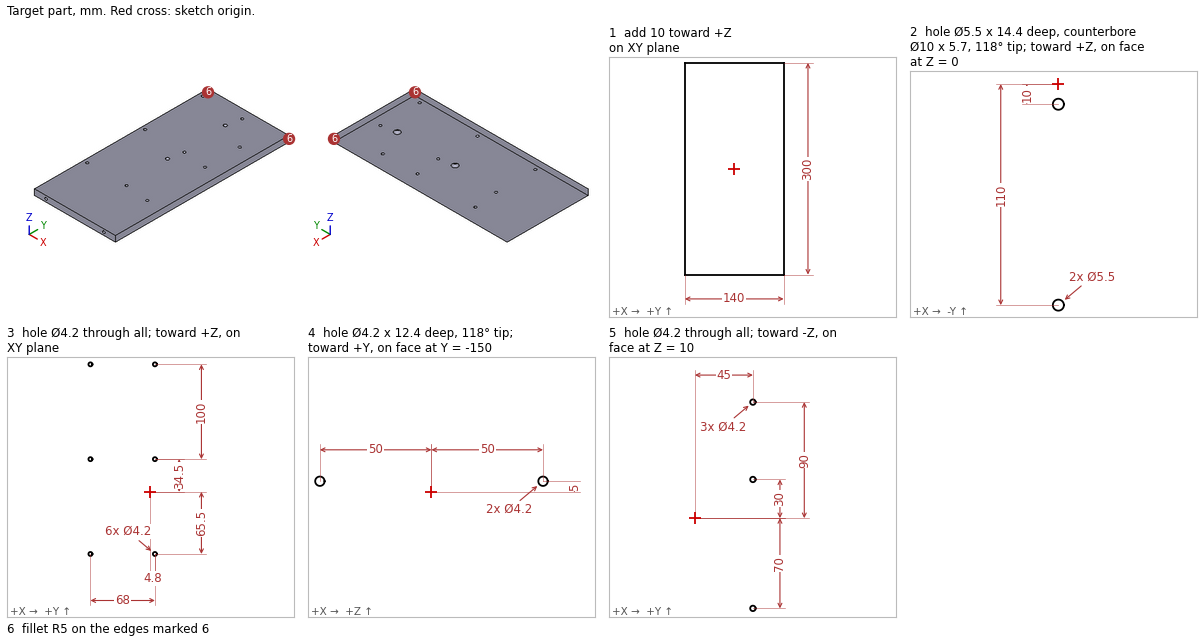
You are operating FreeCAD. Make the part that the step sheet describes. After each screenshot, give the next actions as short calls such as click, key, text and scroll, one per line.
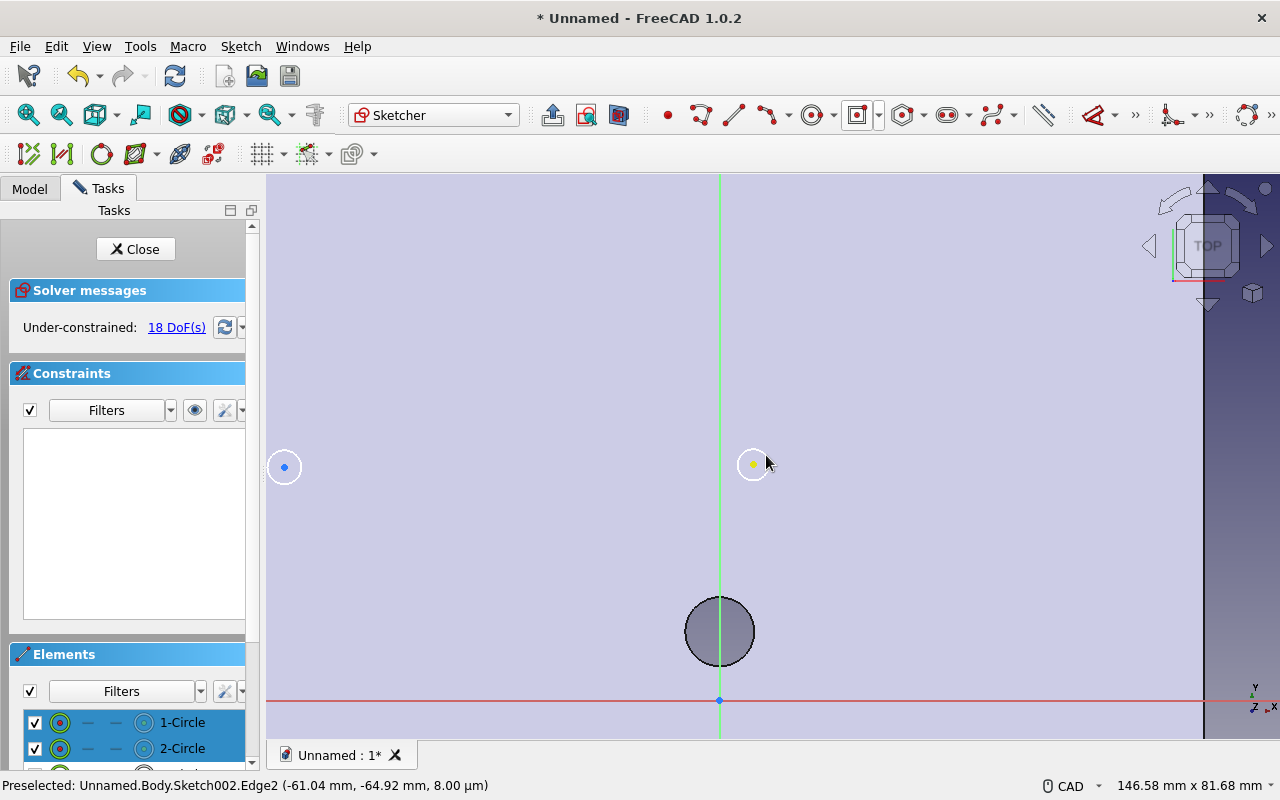
click(764, 454)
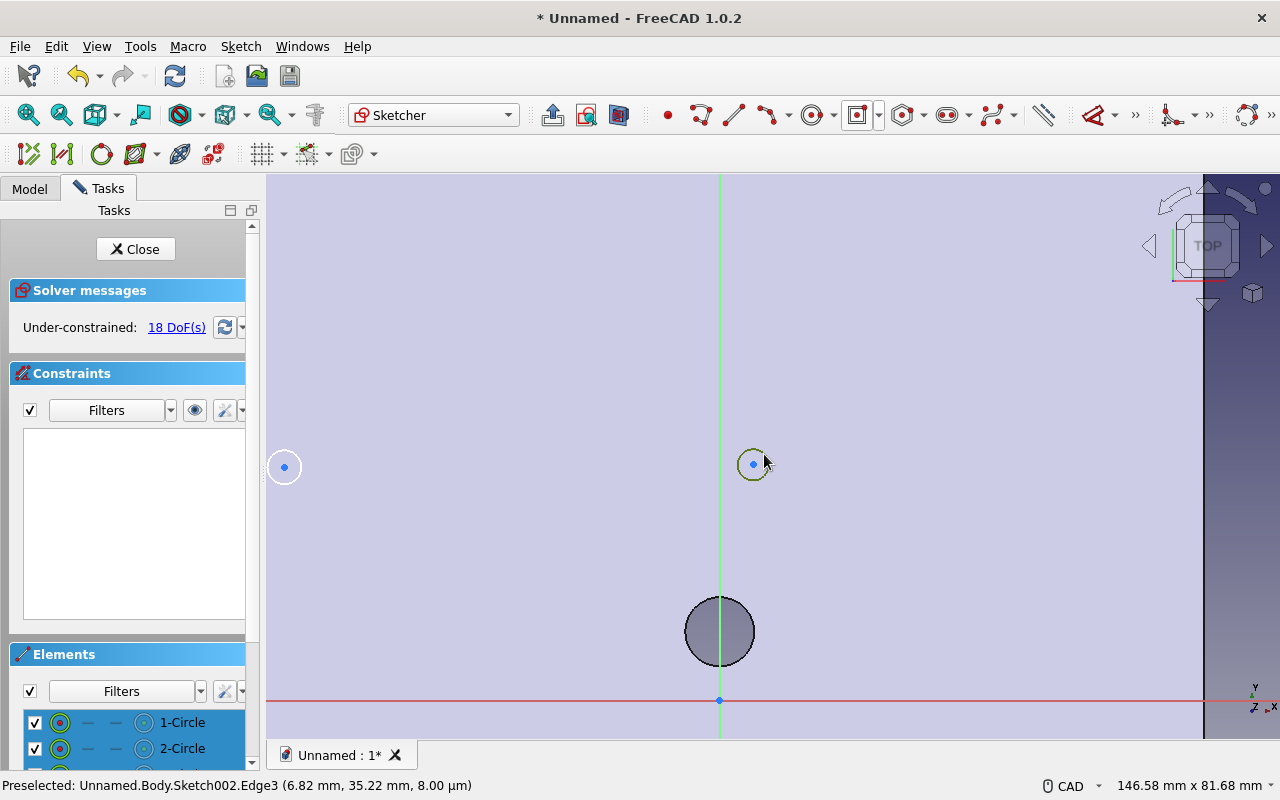
click(296, 455)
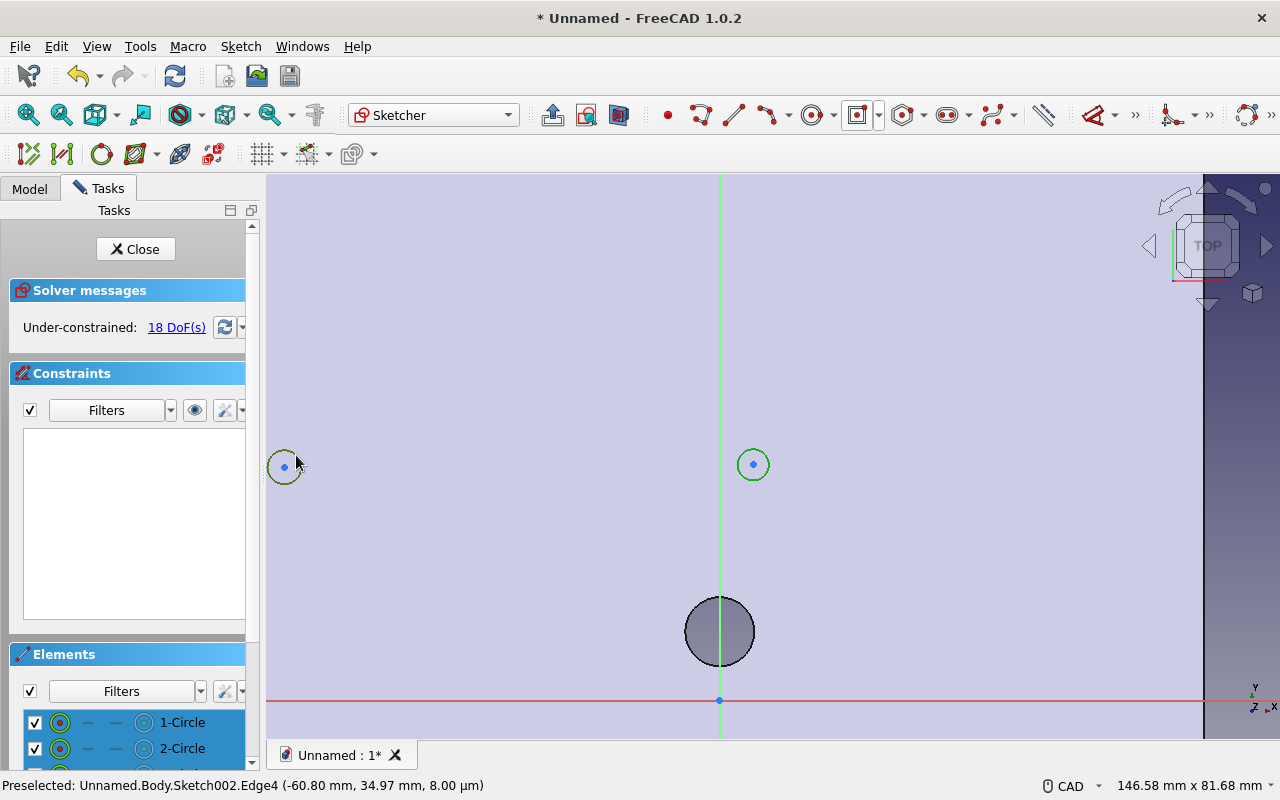
scroll(766, 455, down, 7)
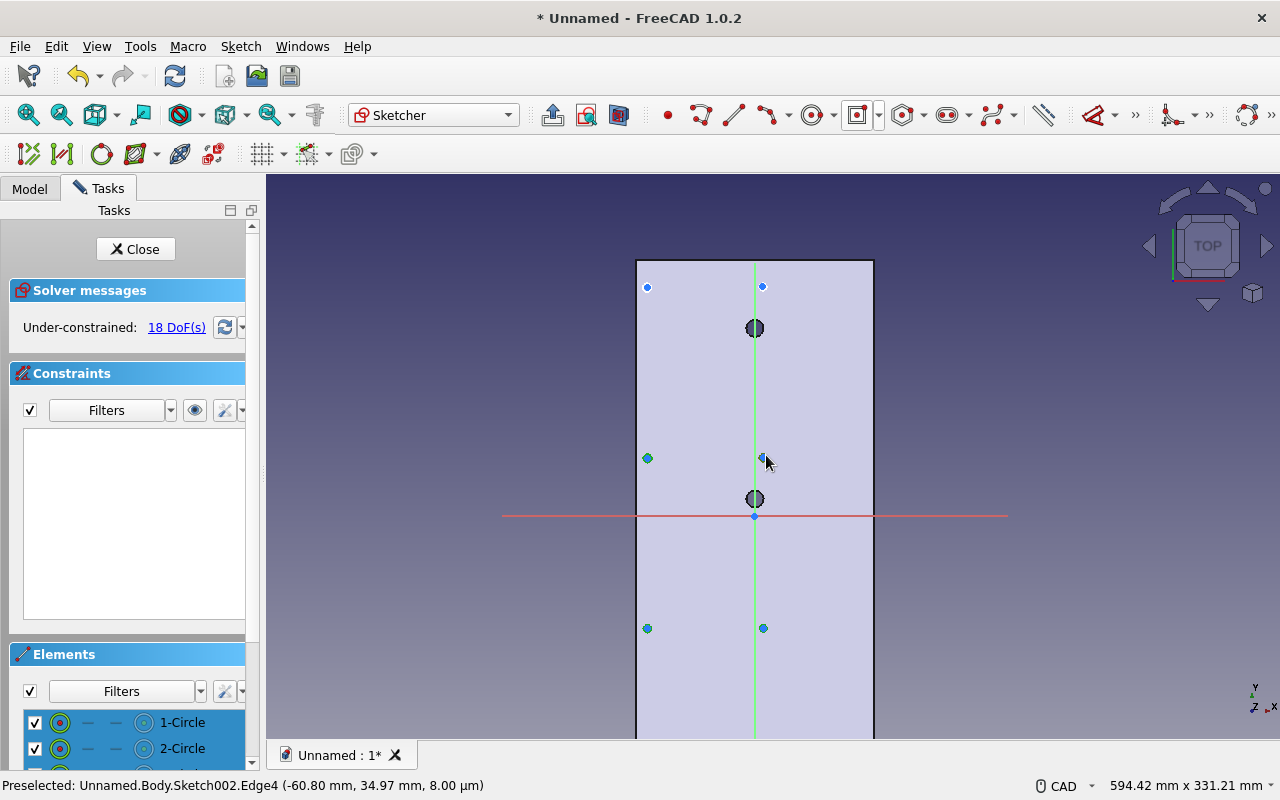
scroll(766, 284, up, 7)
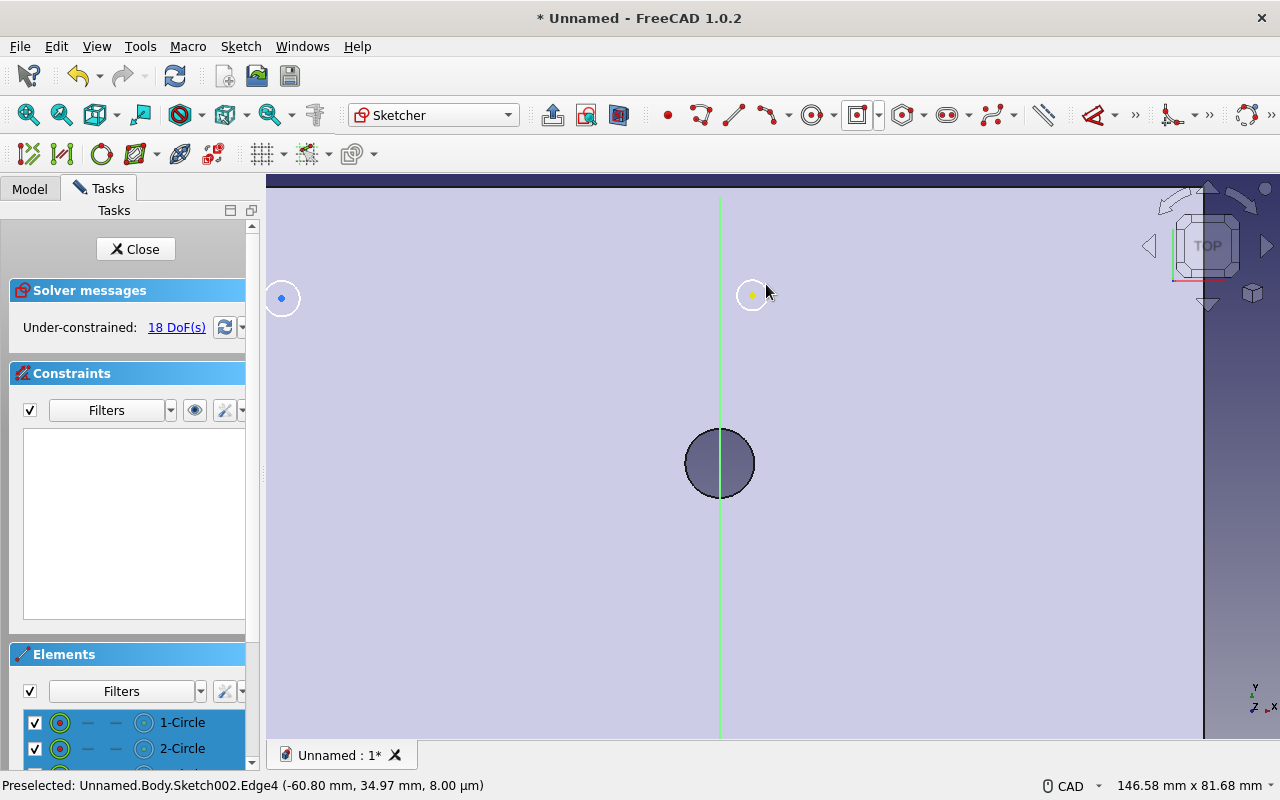
click(763, 285)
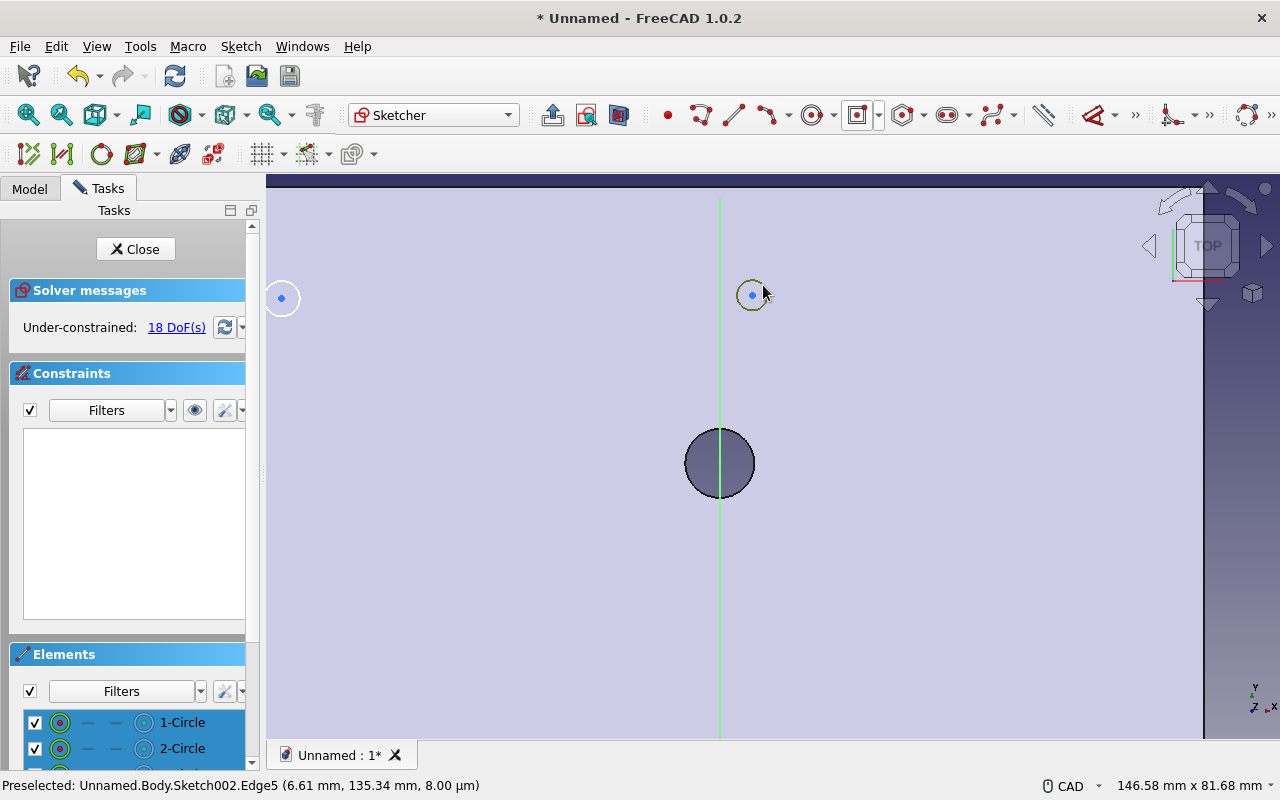
click(294, 286)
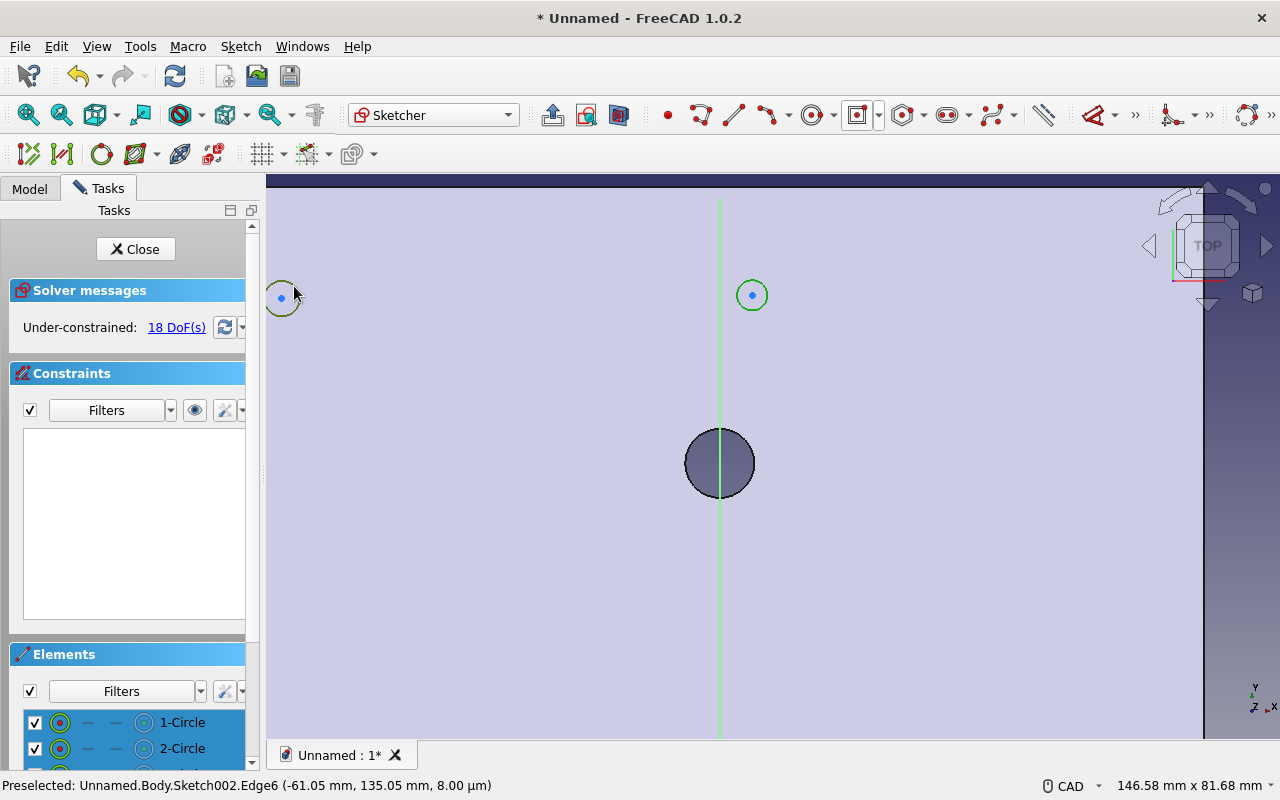
key(e)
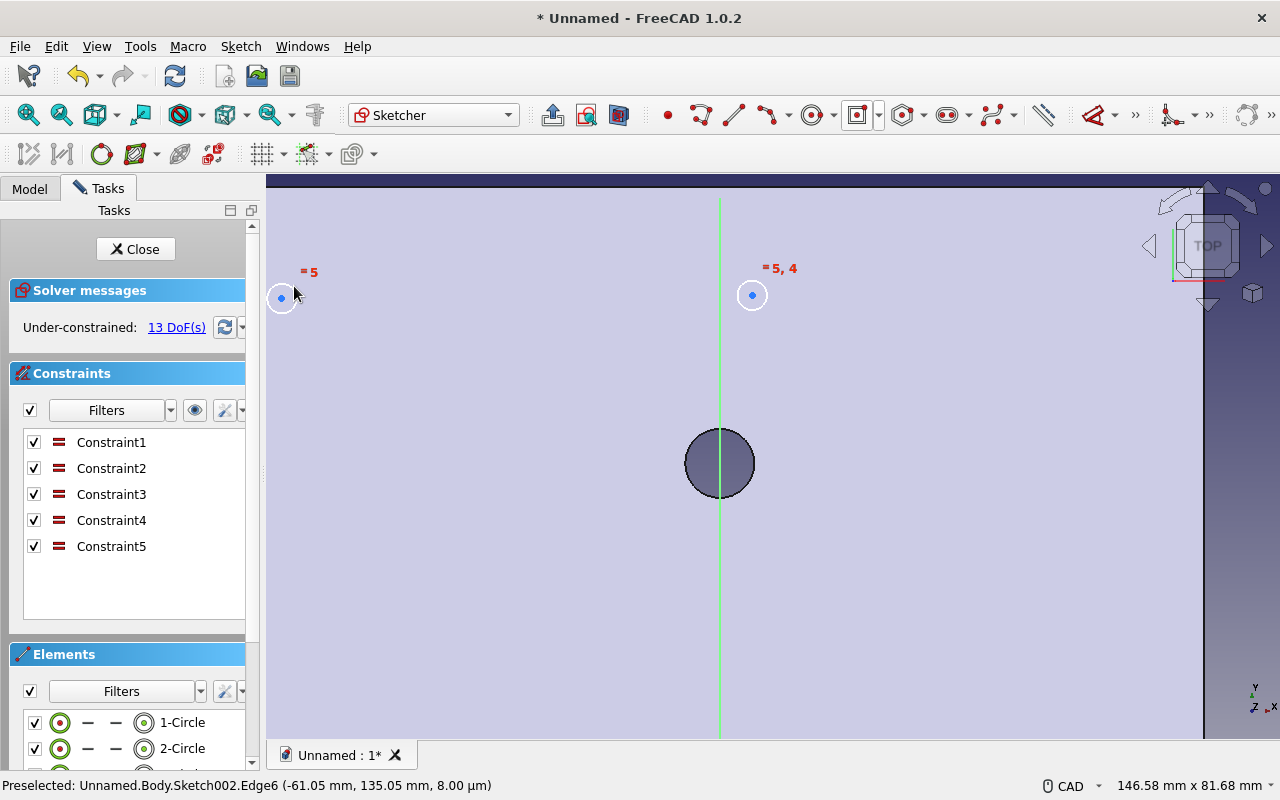
scroll(766, 283, down, 7)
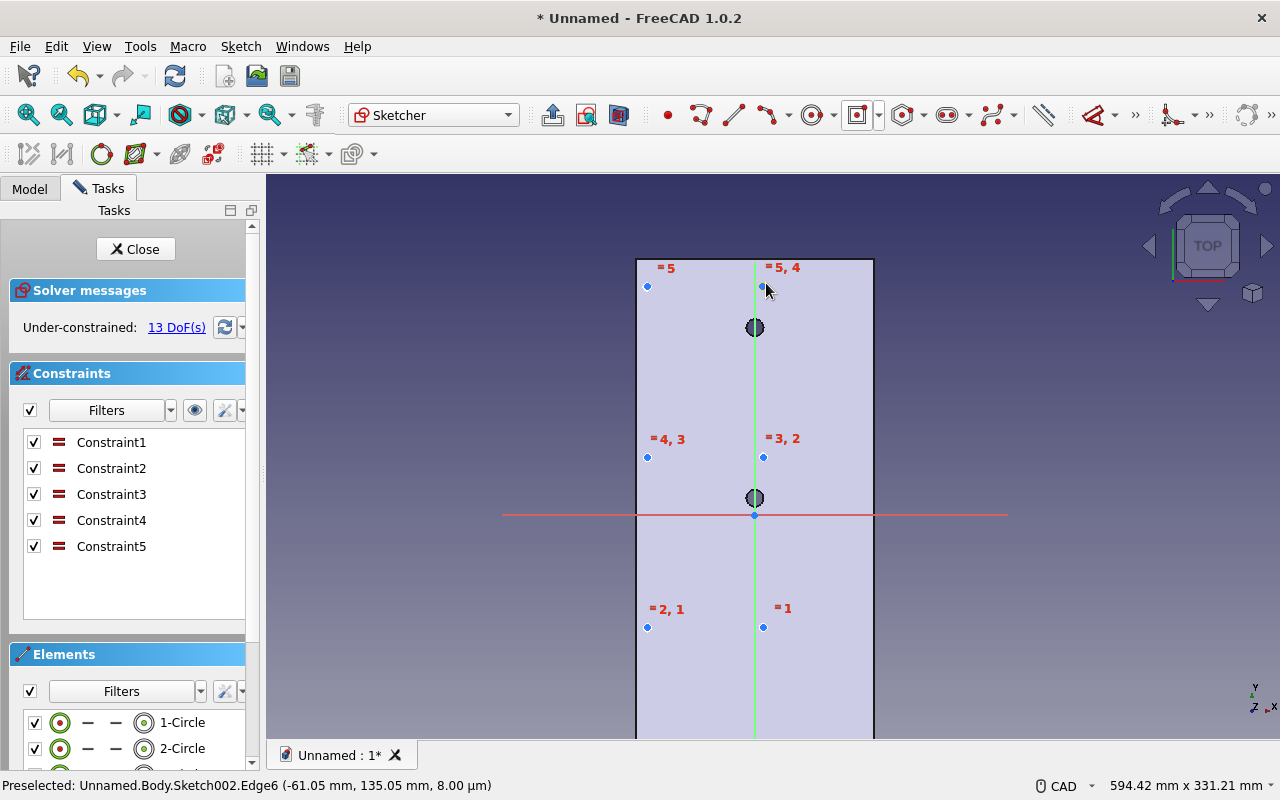
click(763, 627)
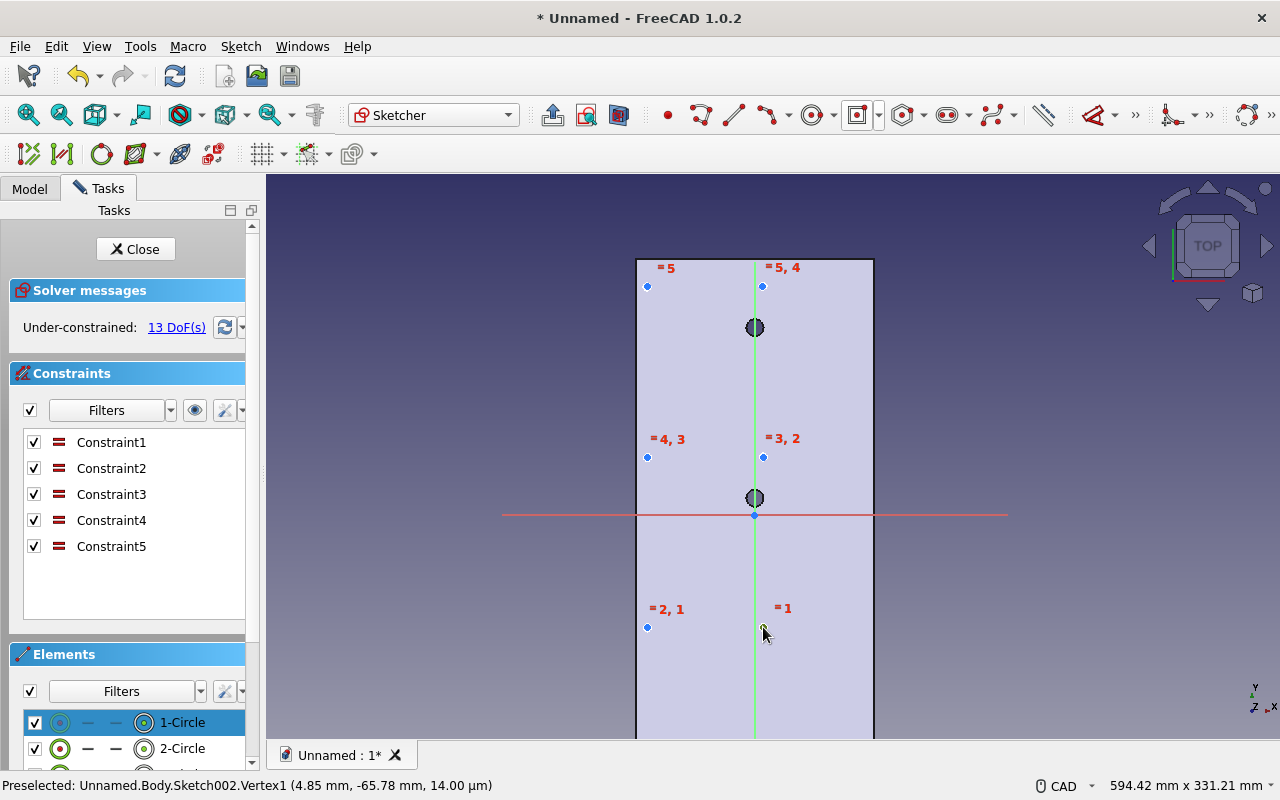
click(647, 628)